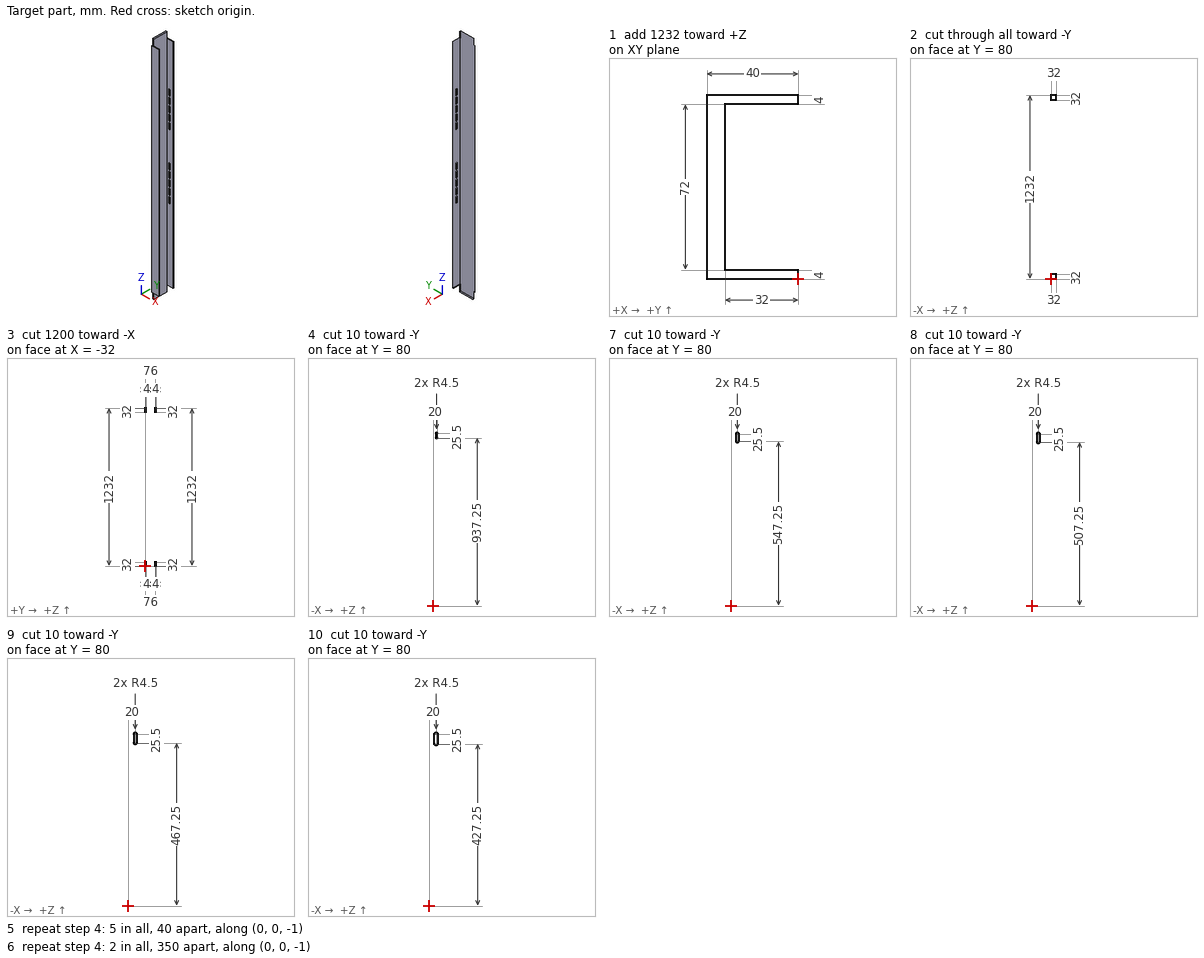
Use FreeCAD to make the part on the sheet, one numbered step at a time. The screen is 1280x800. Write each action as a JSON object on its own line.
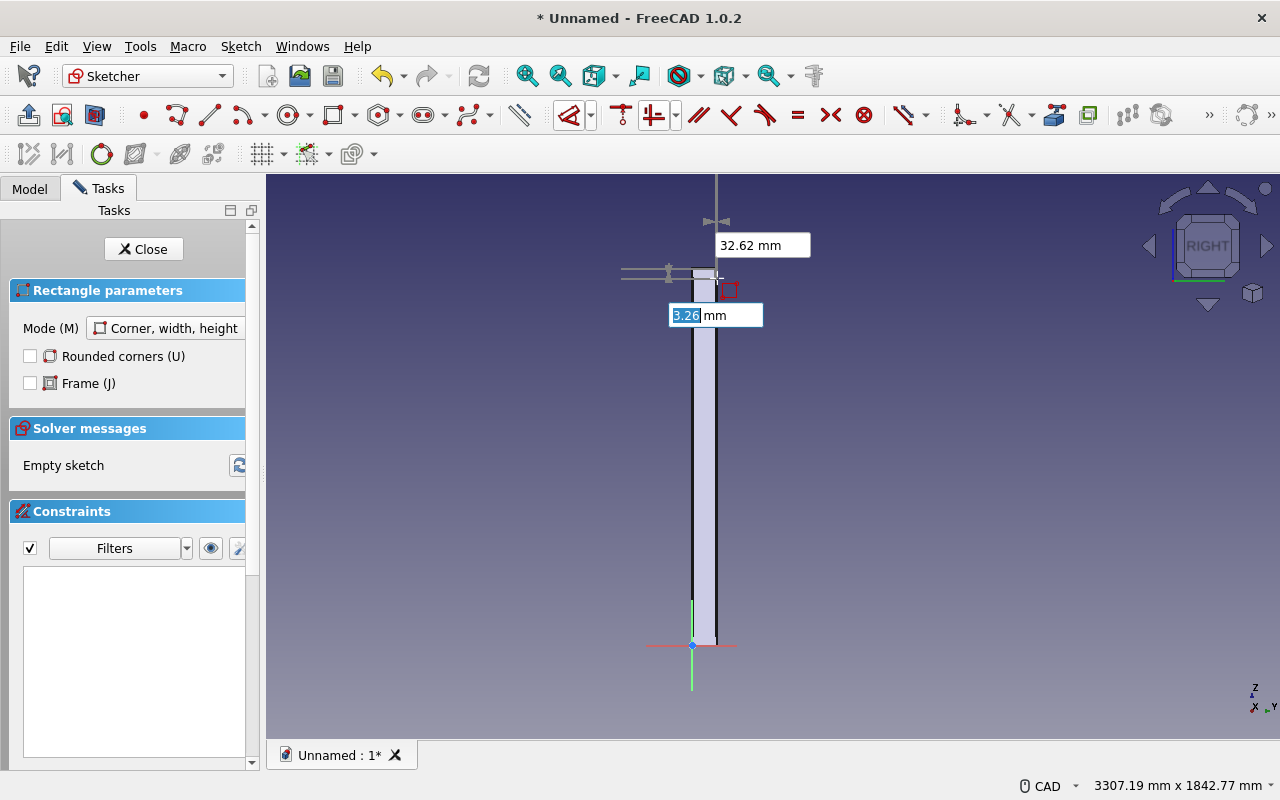
{"action": "type", "text": "4"}
{"action": "key", "text": "Tab"}
{"action": "type", "text": "32"}
{"action": "key", "text": "Return"}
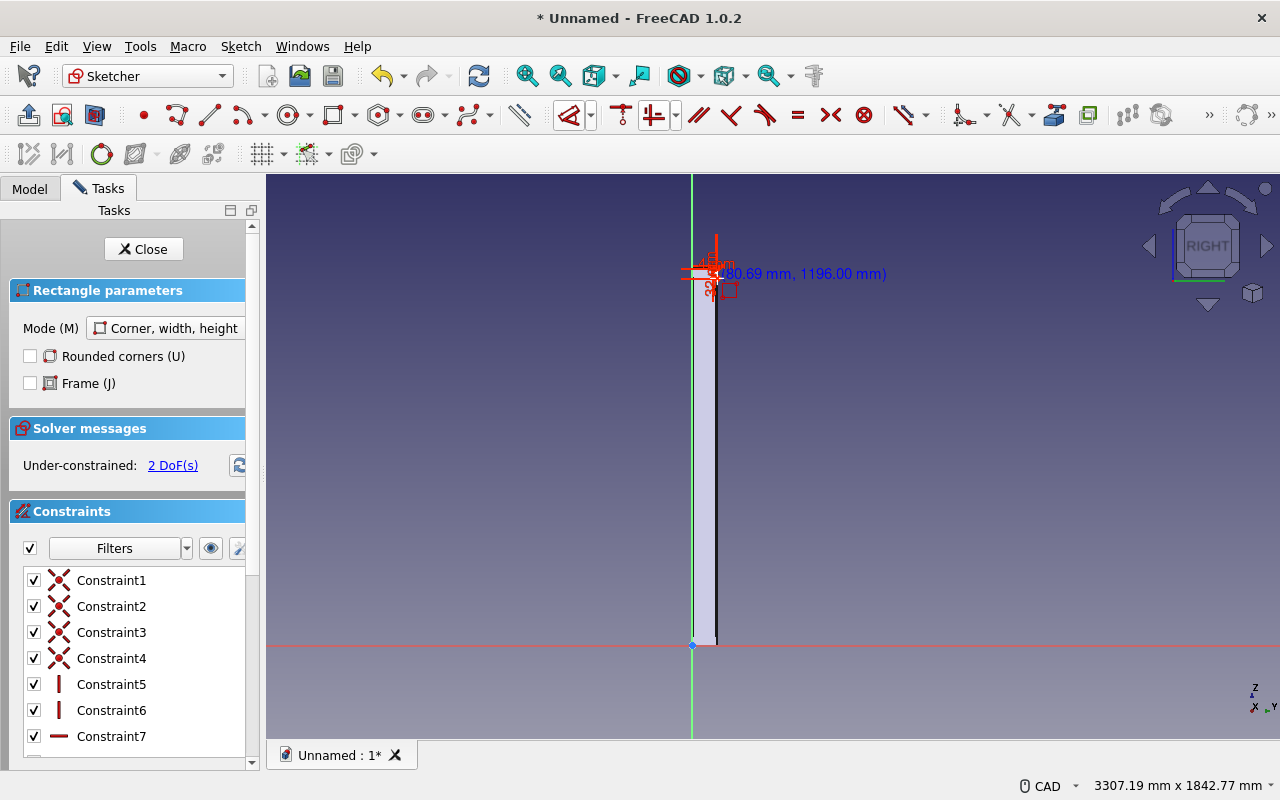
{"action": "scroll", "coordinate": [692, 268], "scroll_direction": "up", "scroll_amount": 13}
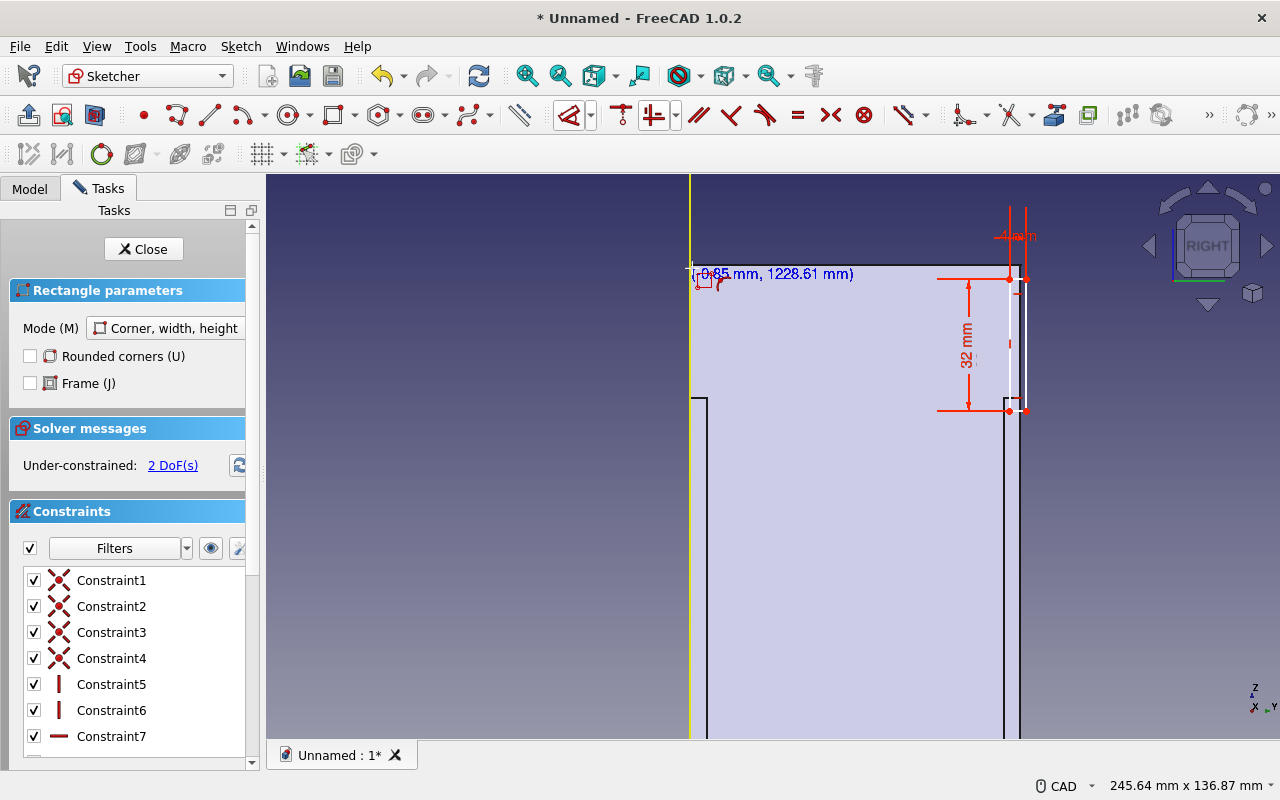
{"action": "scroll", "coordinate": [692, 268], "scroll_direction": "down", "scroll_amount": 13}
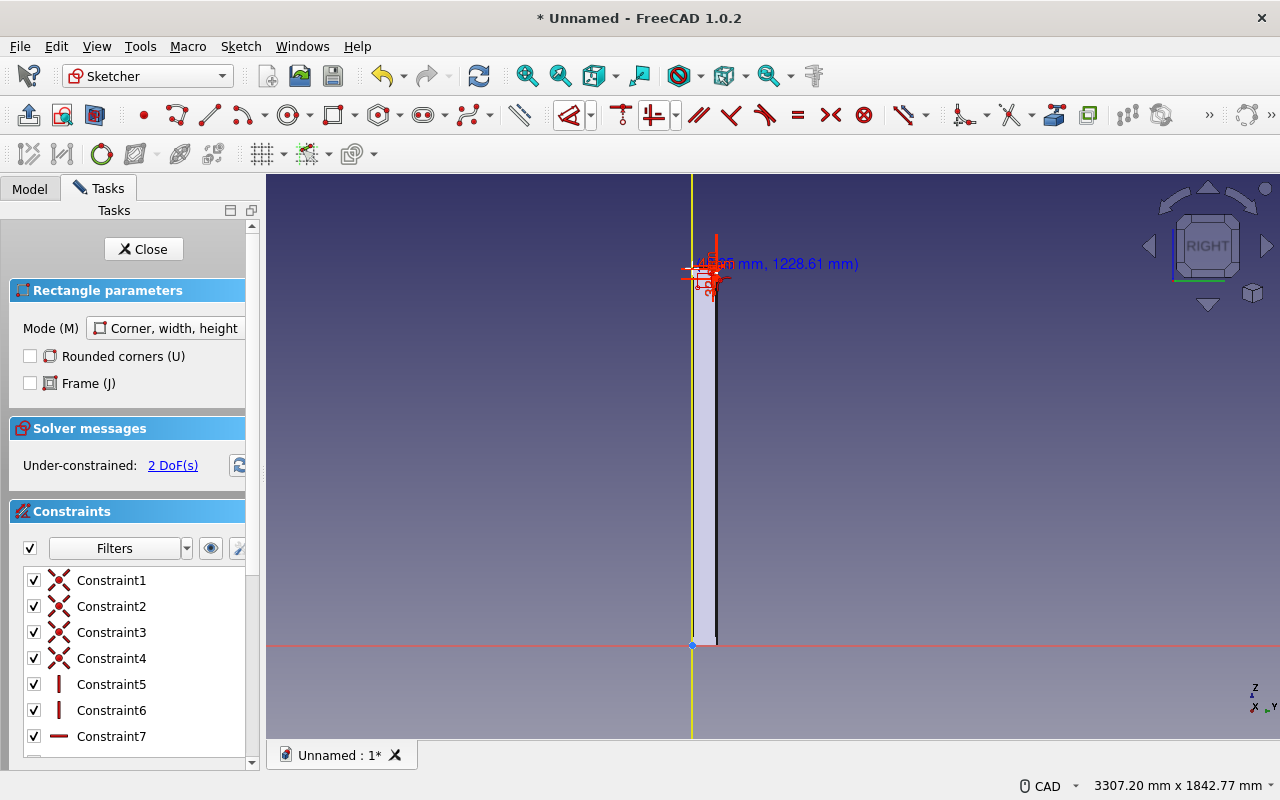
{"action": "left_click", "coordinate": [692, 268]}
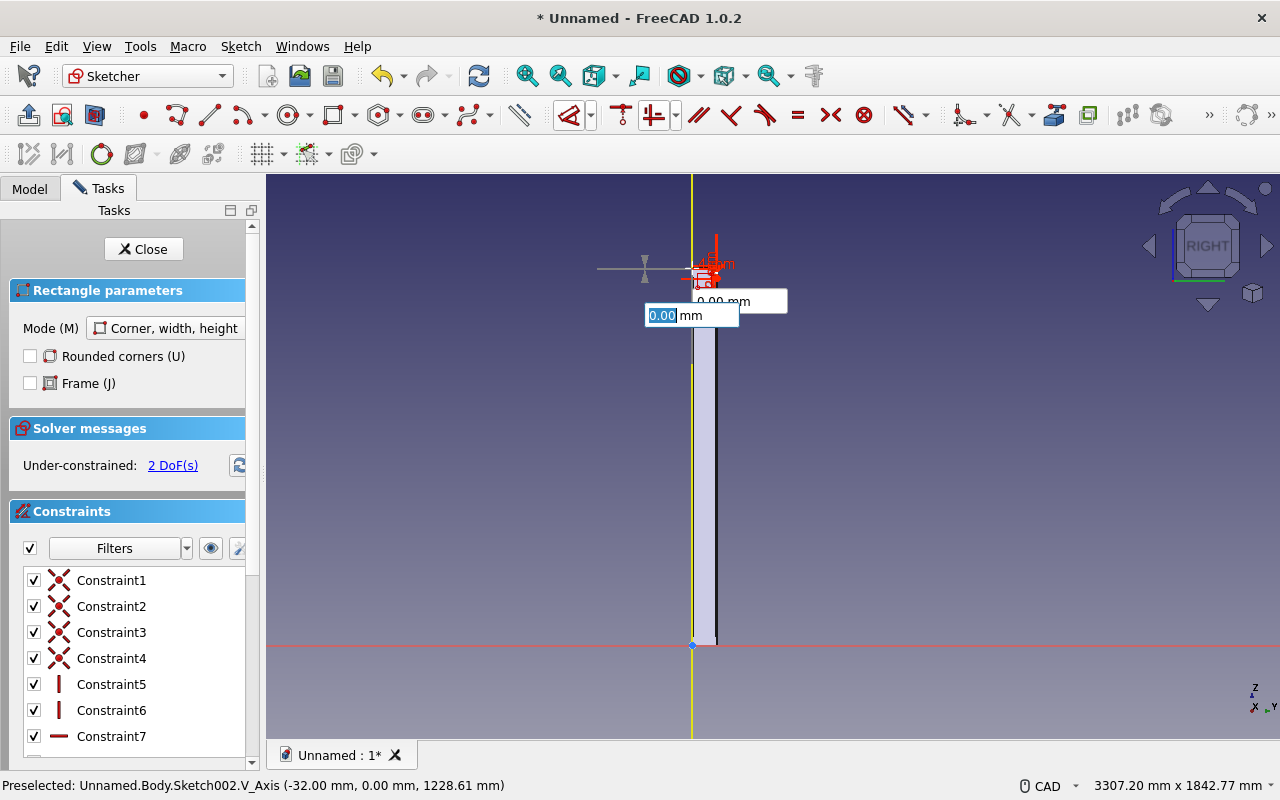
{"action": "scroll", "coordinate": [693, 278], "scroll_direction": "up", "scroll_amount": 13}
{"action": "mouse_move", "coordinate": [694, 273]}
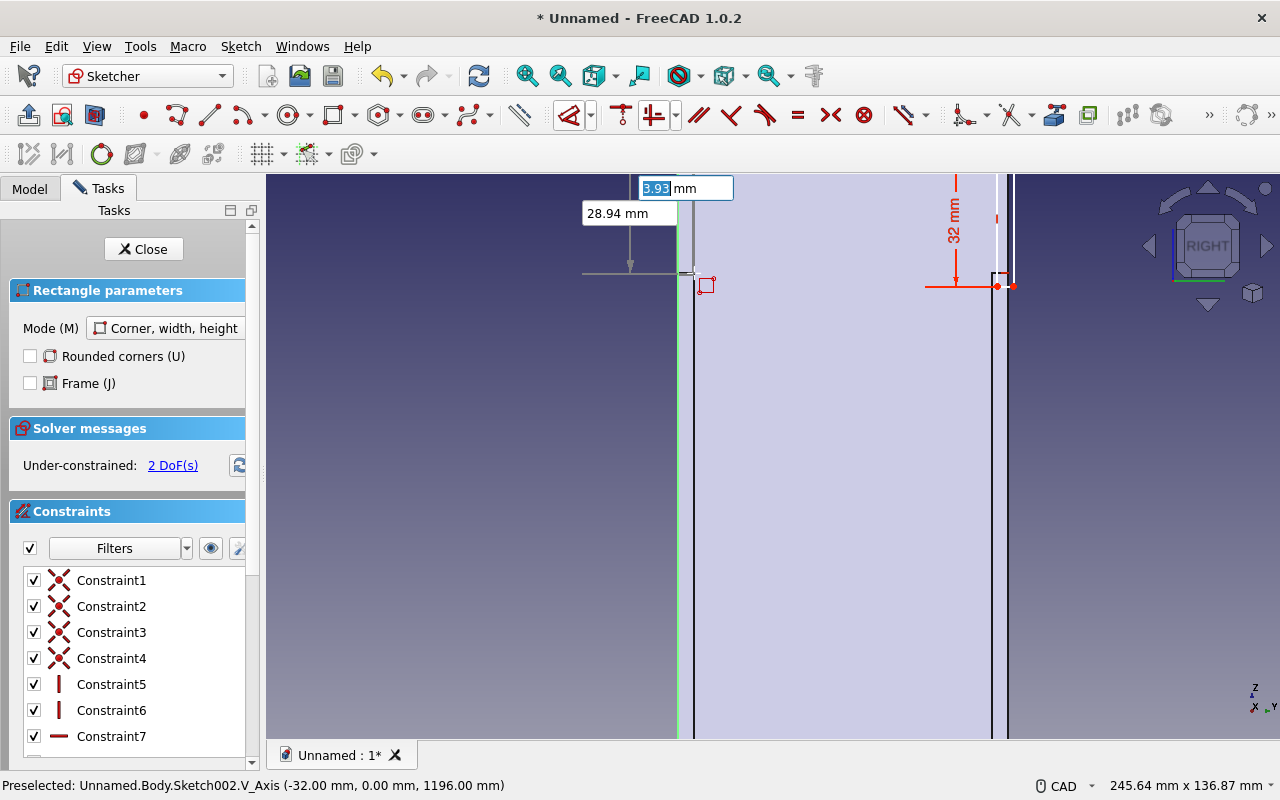
{"action": "type", "text": "4"}
{"action": "key", "text": "Tab"}
{"action": "type", "text": "32"}
{"action": "key", "text": "Return"}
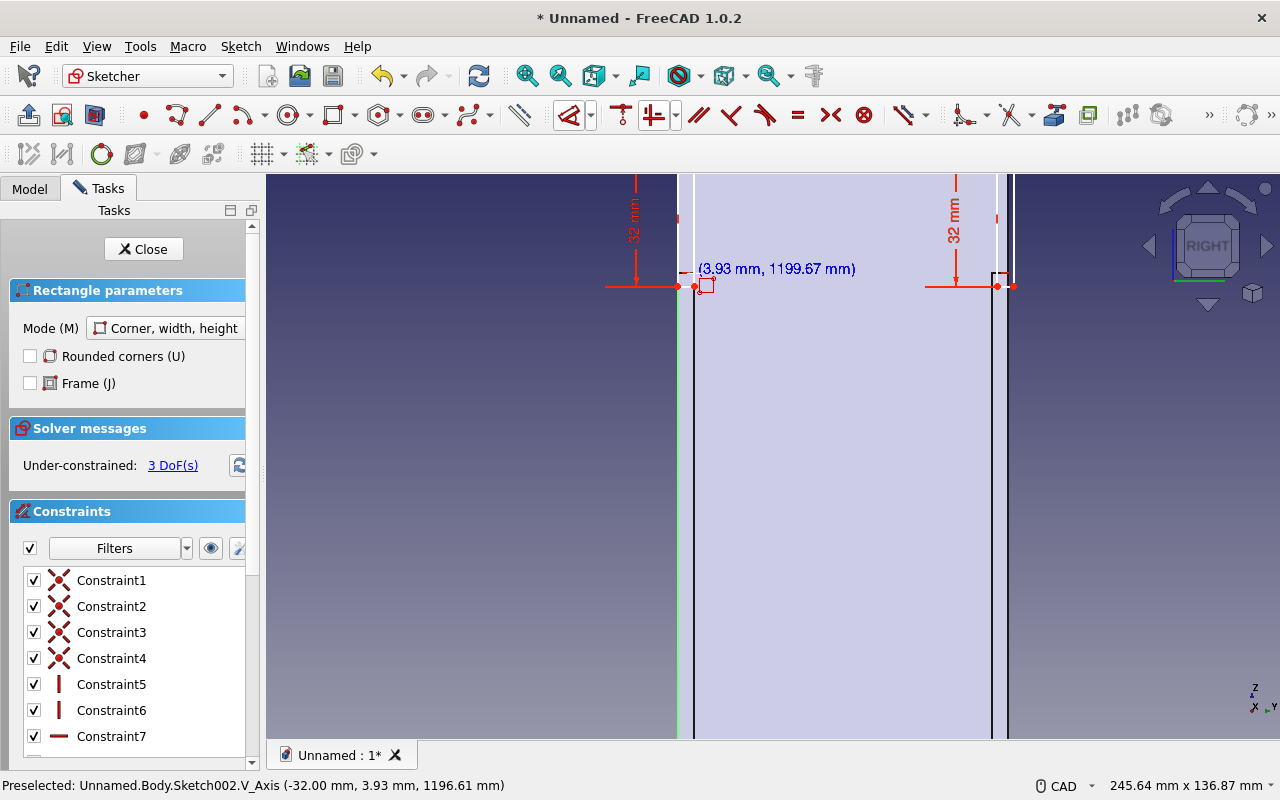
{"action": "scroll", "coordinate": [693, 278], "scroll_direction": "down", "scroll_amount": 13}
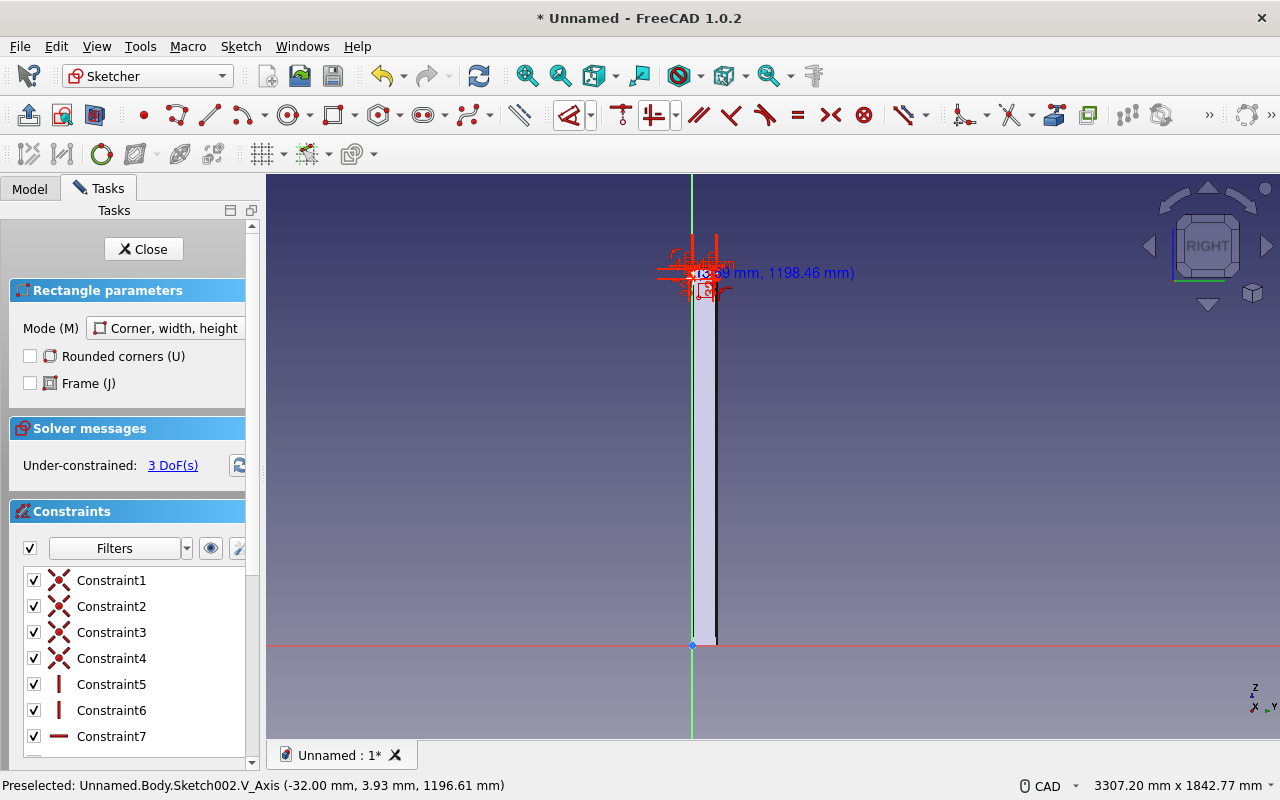
{"action": "scroll", "coordinate": [716, 636], "scroll_direction": "up", "scroll_amount": 13}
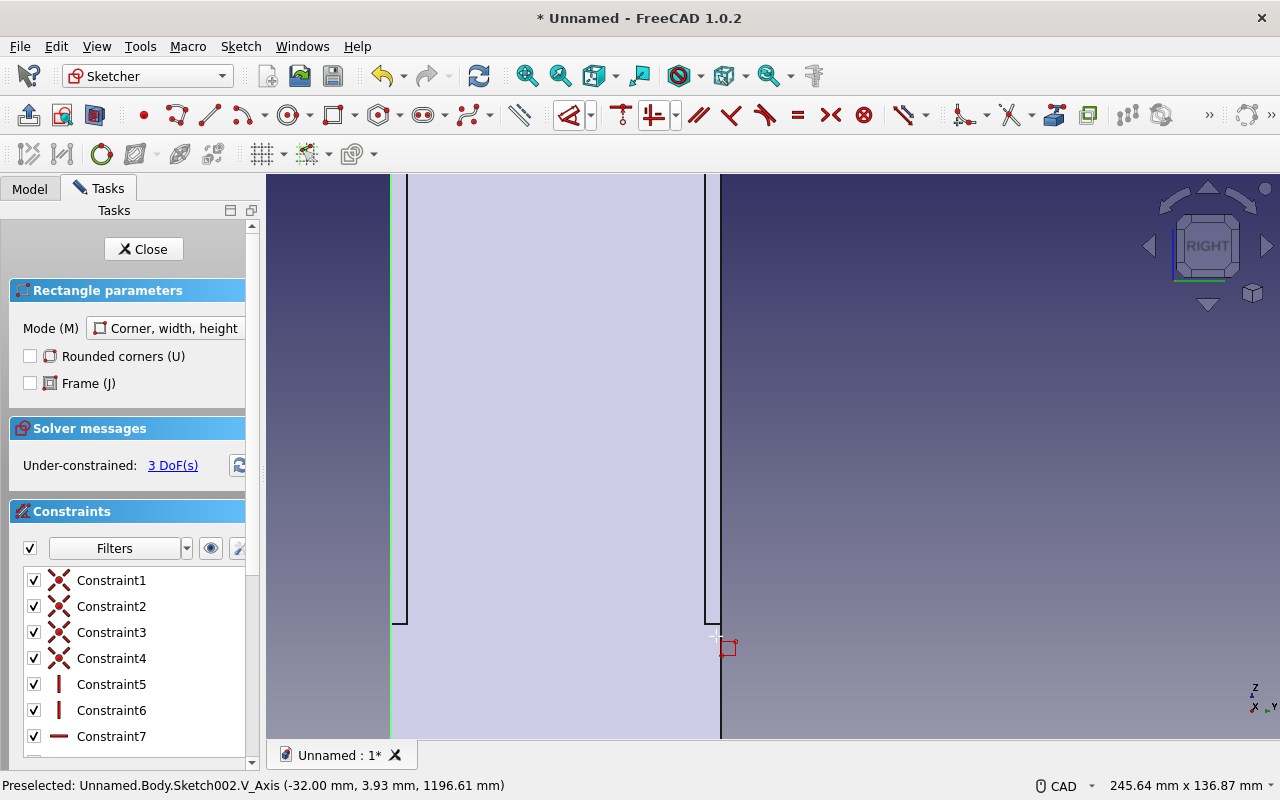
{"action": "scroll", "coordinate": [716, 636], "scroll_direction": "down", "scroll_amount": 13}